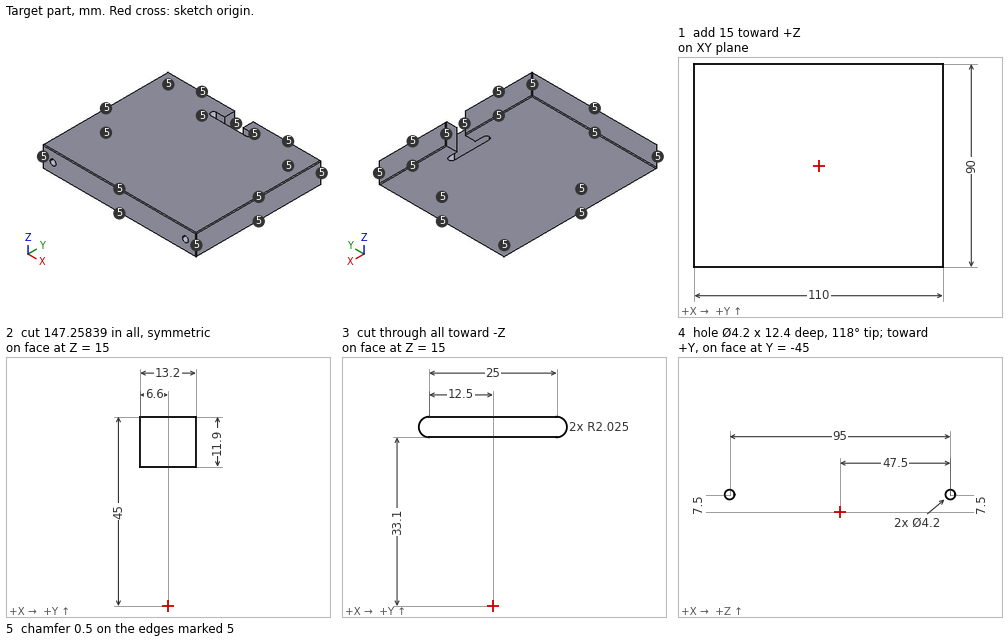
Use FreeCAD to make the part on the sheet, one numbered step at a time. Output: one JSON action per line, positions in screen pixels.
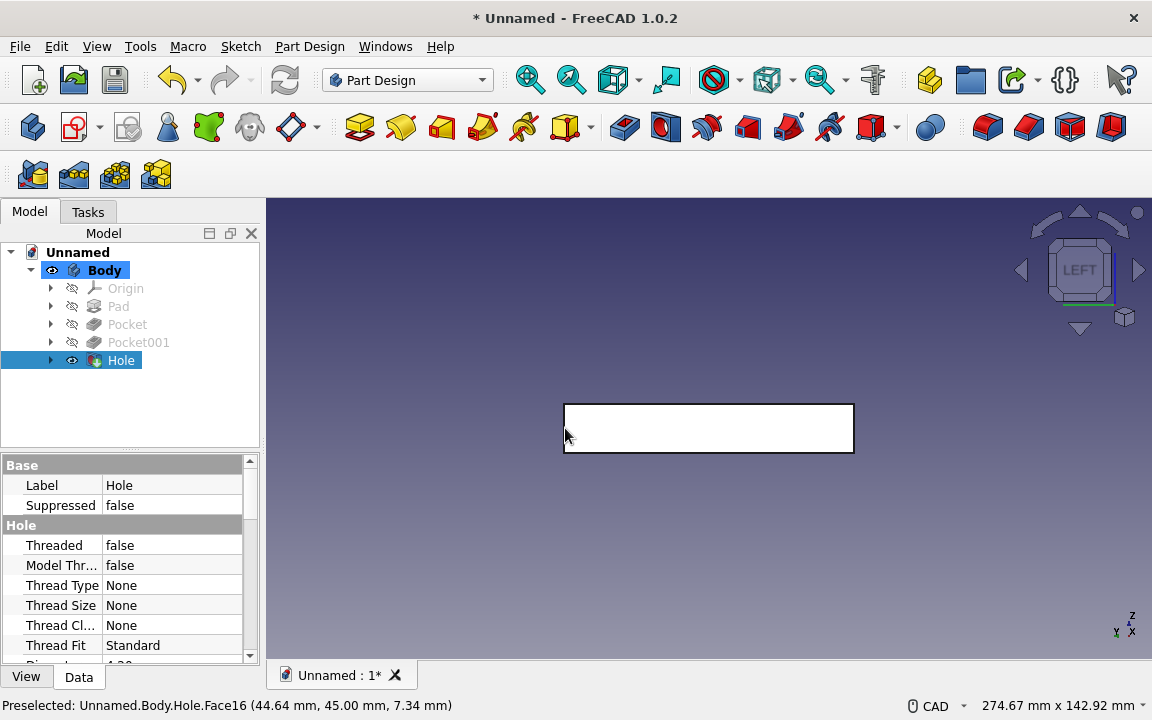
{"action": "left_click", "coordinate": [531, 80]}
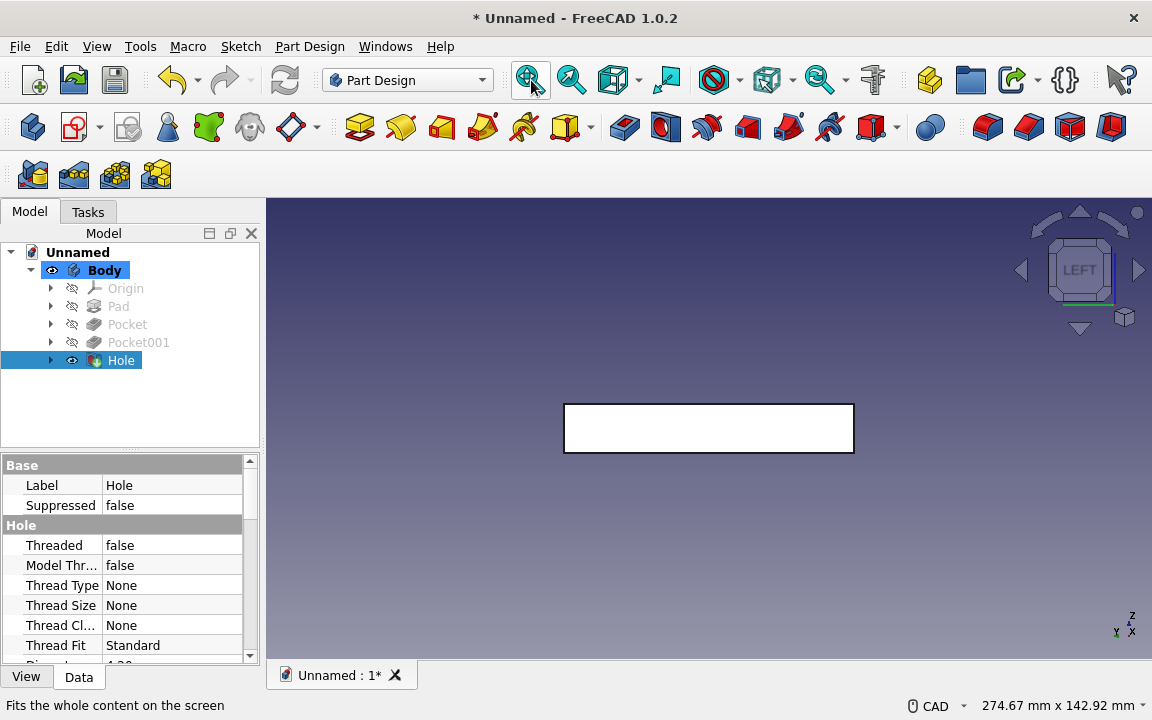
{"action": "left_click", "coordinate": [626, 427], "text": "ctrl"}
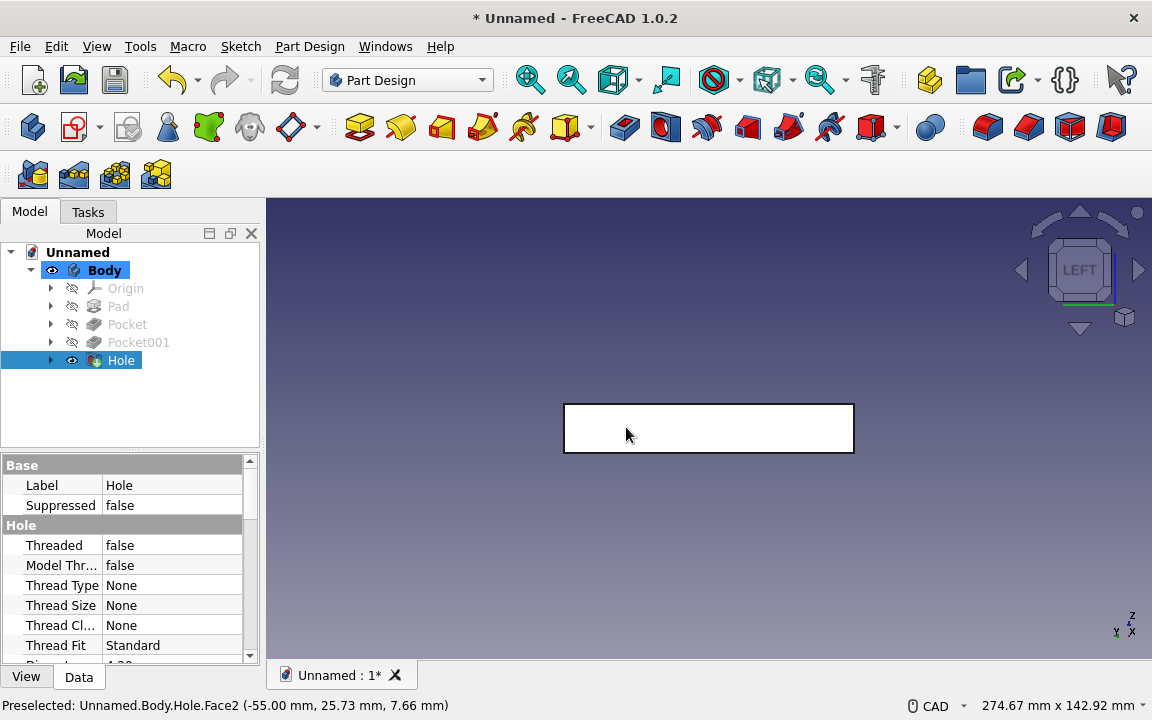
{"action": "left_click", "coordinate": [1029, 128]}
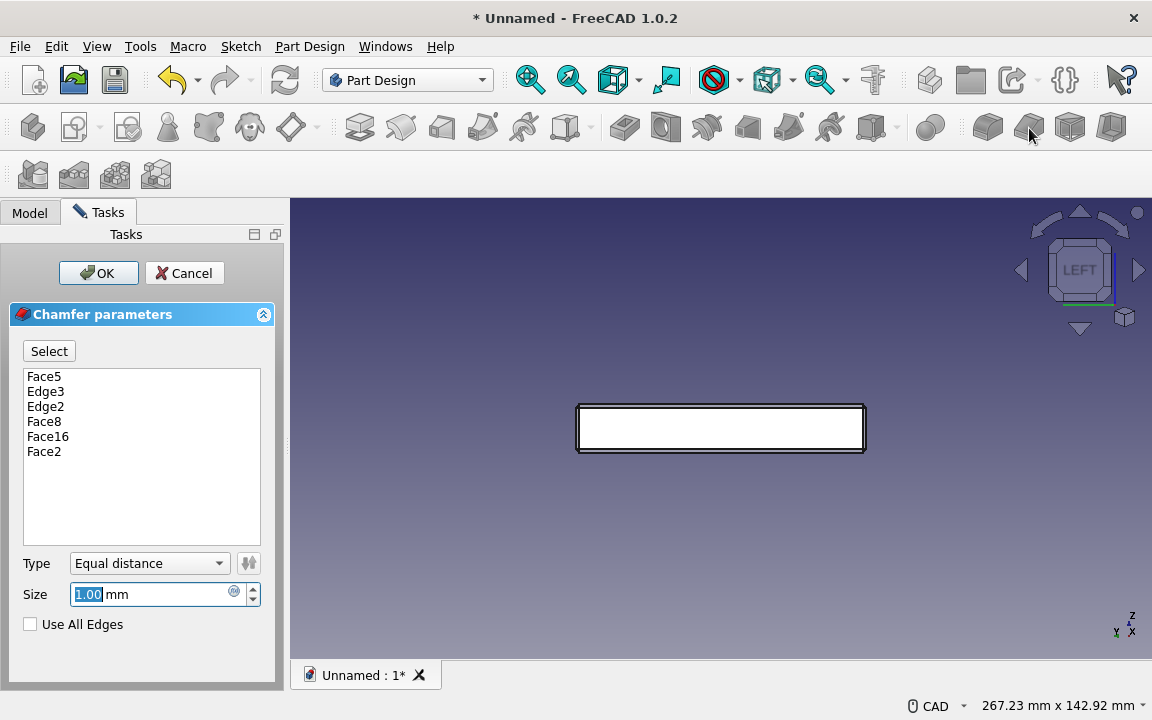
{"action": "type", "text": "0.5"}
{"action": "key", "text": "Tab"}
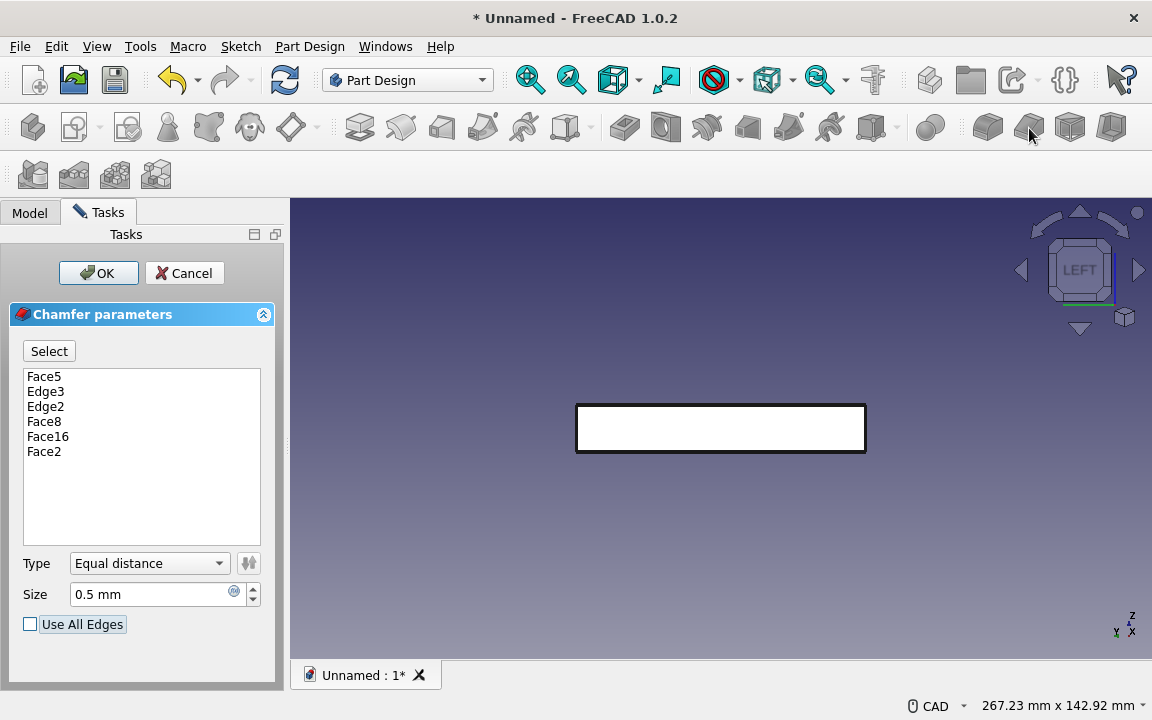
{"action": "left_click", "coordinate": [99, 273]}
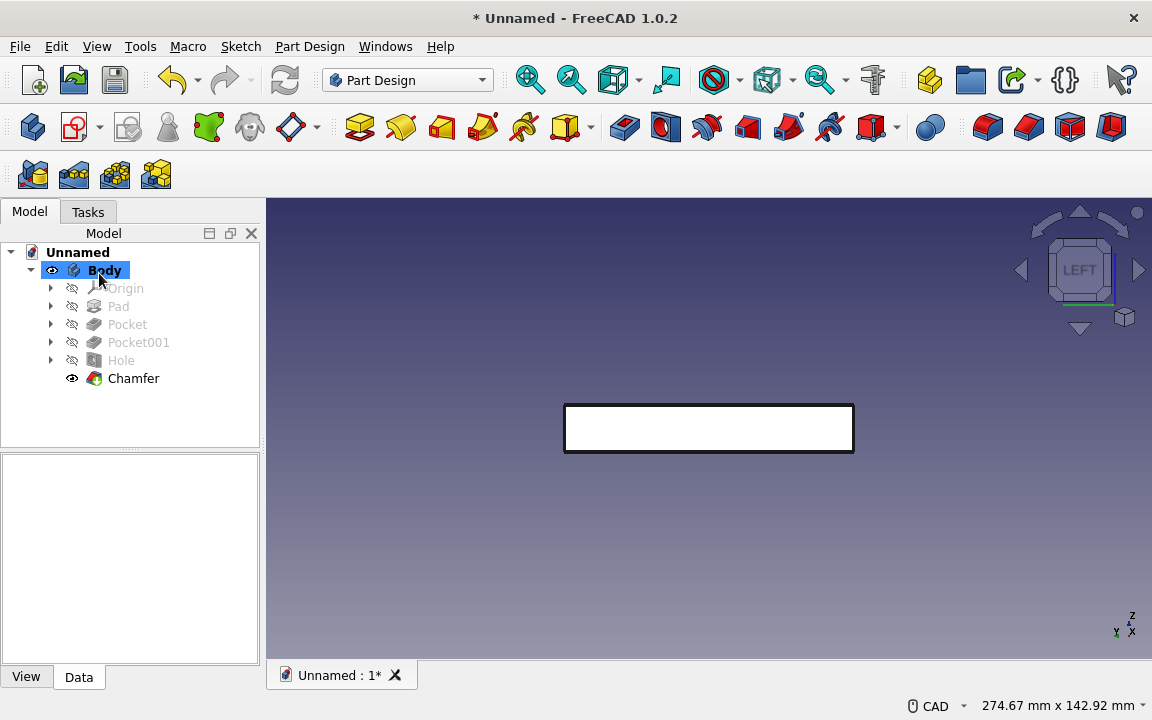
{"action": "key", "text": "0"}